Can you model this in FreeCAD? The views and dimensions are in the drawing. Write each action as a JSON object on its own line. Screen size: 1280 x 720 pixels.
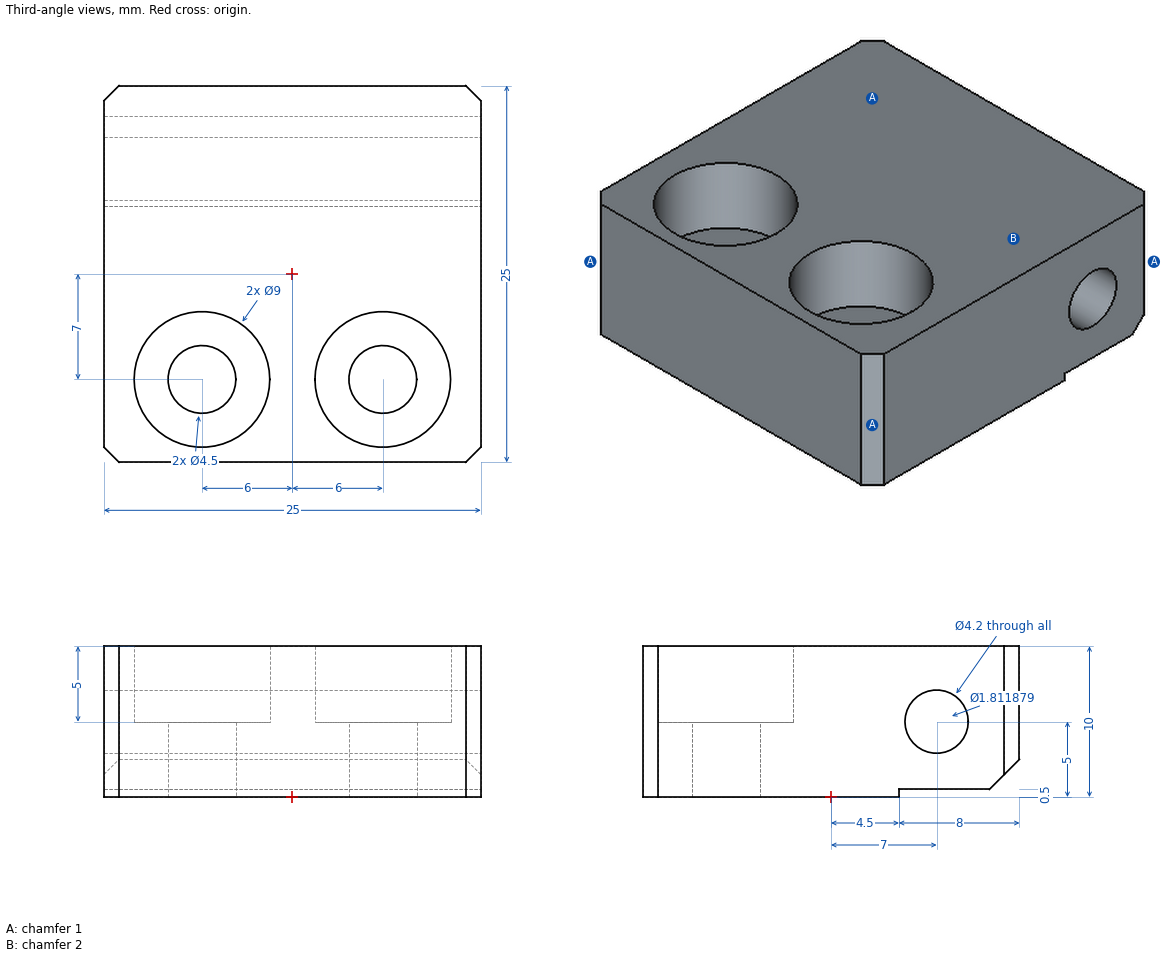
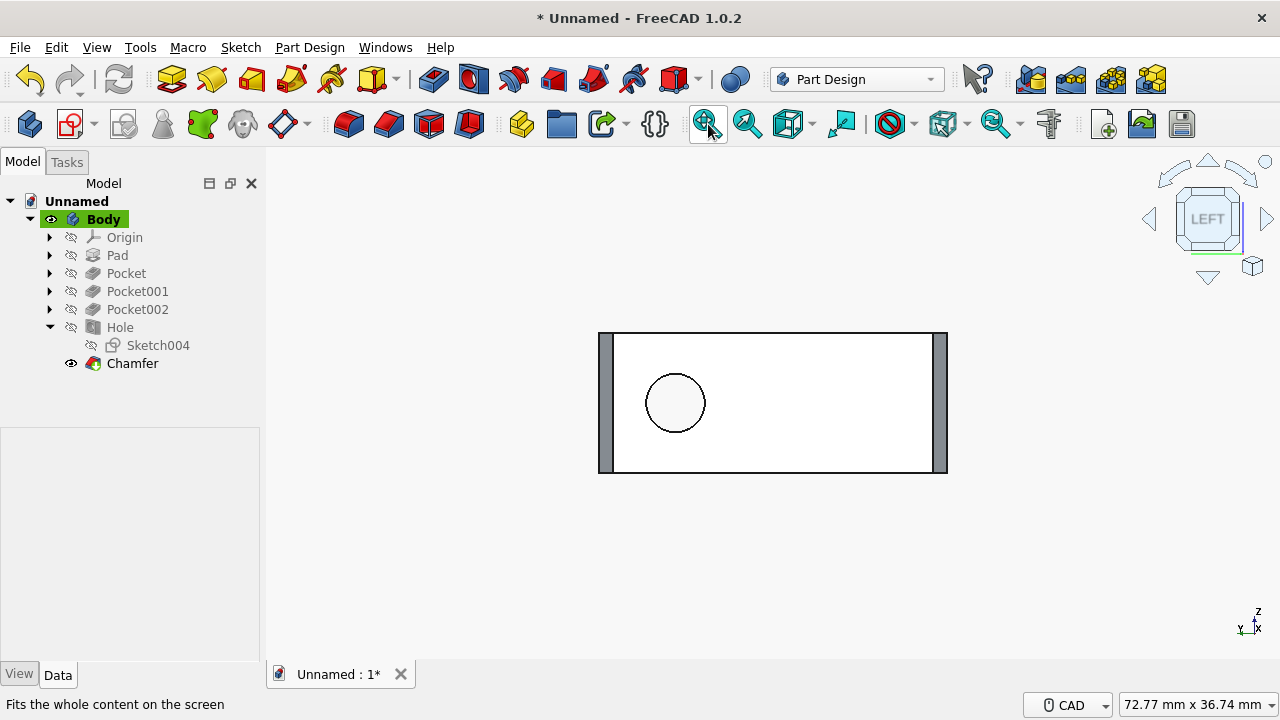
{"action": "left_click", "coordinate": [708, 124]}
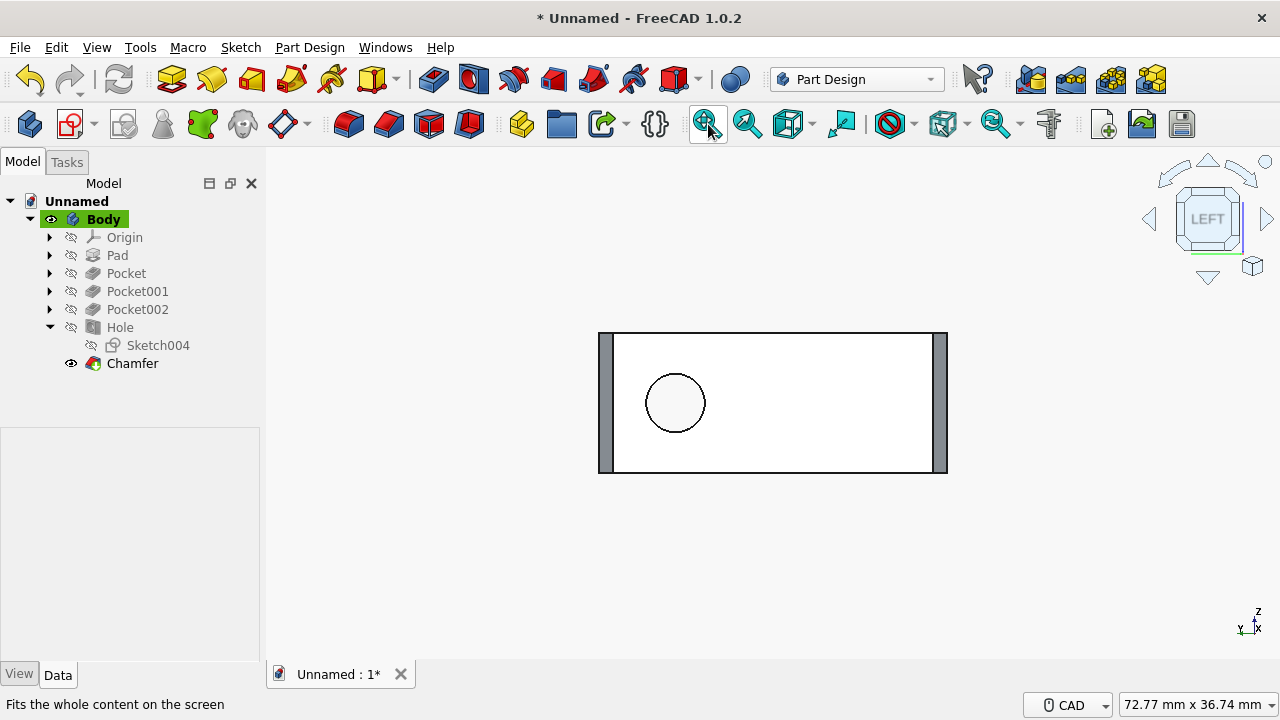
{"action": "left_click", "coordinate": [819, 402]}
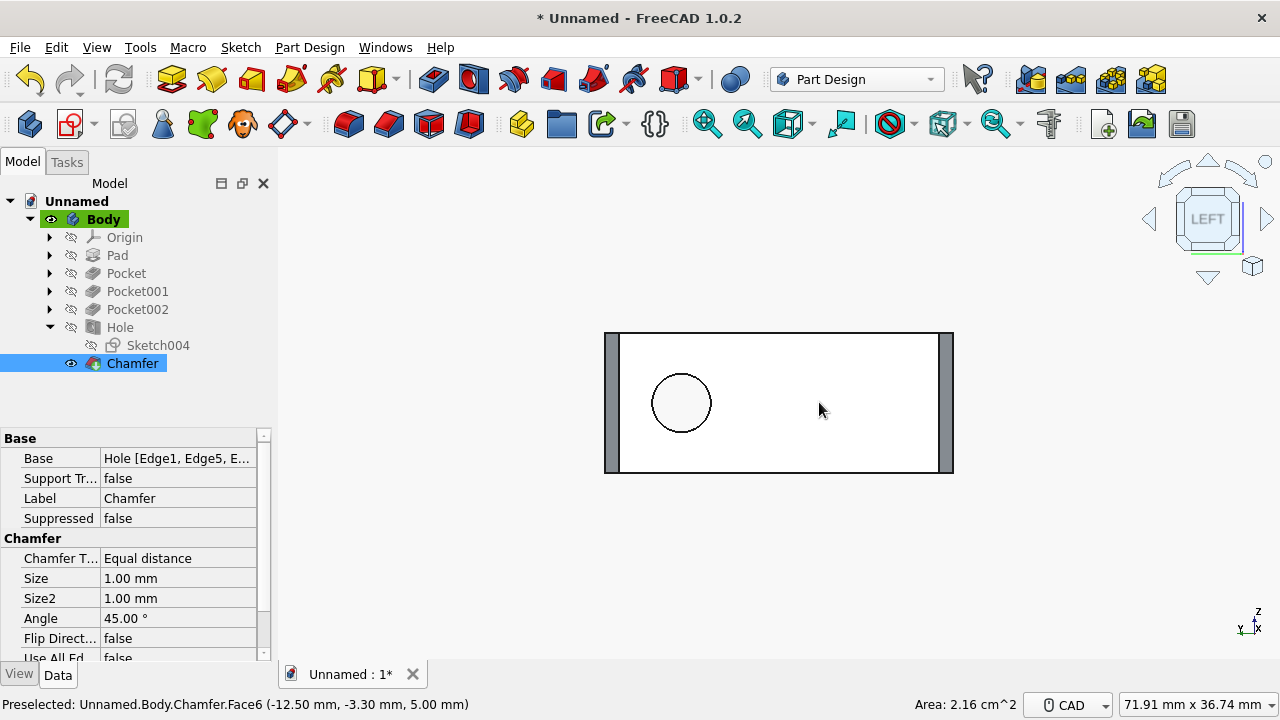
{"action": "left_click", "coordinate": [70, 124]}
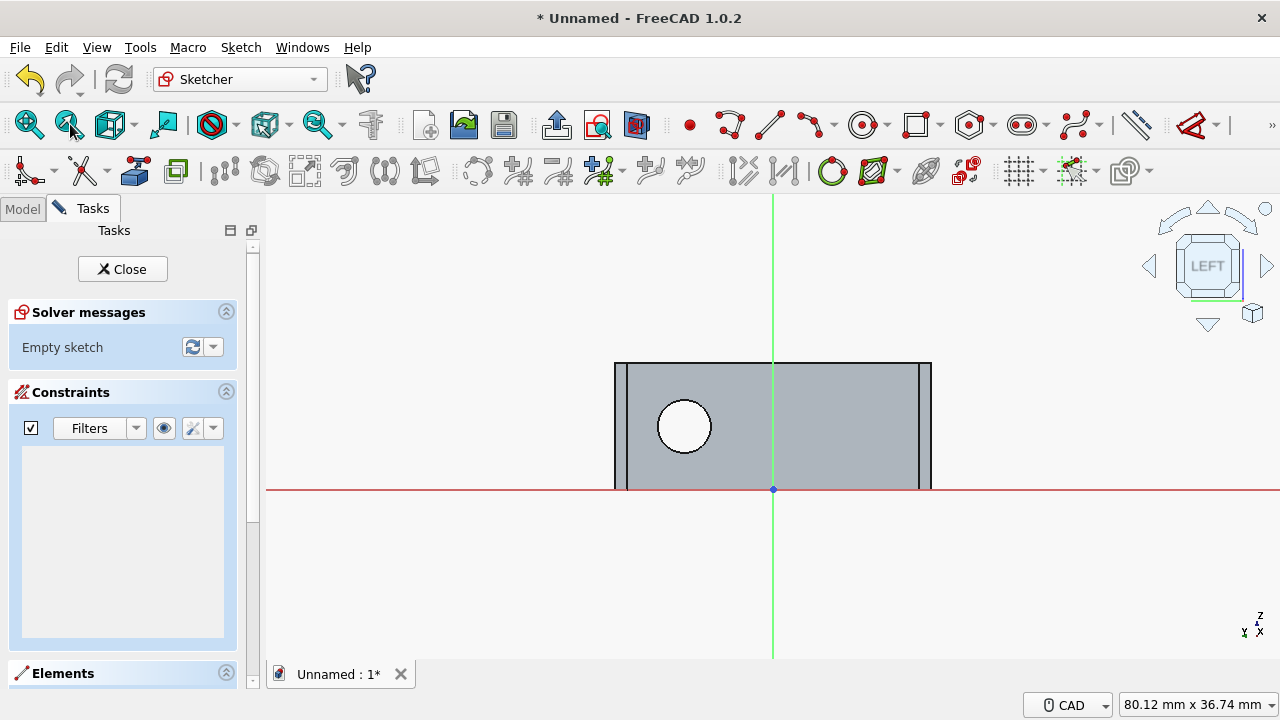
{"action": "scroll", "coordinate": [689, 513], "scroll_direction": "up", "scroll_amount": 6}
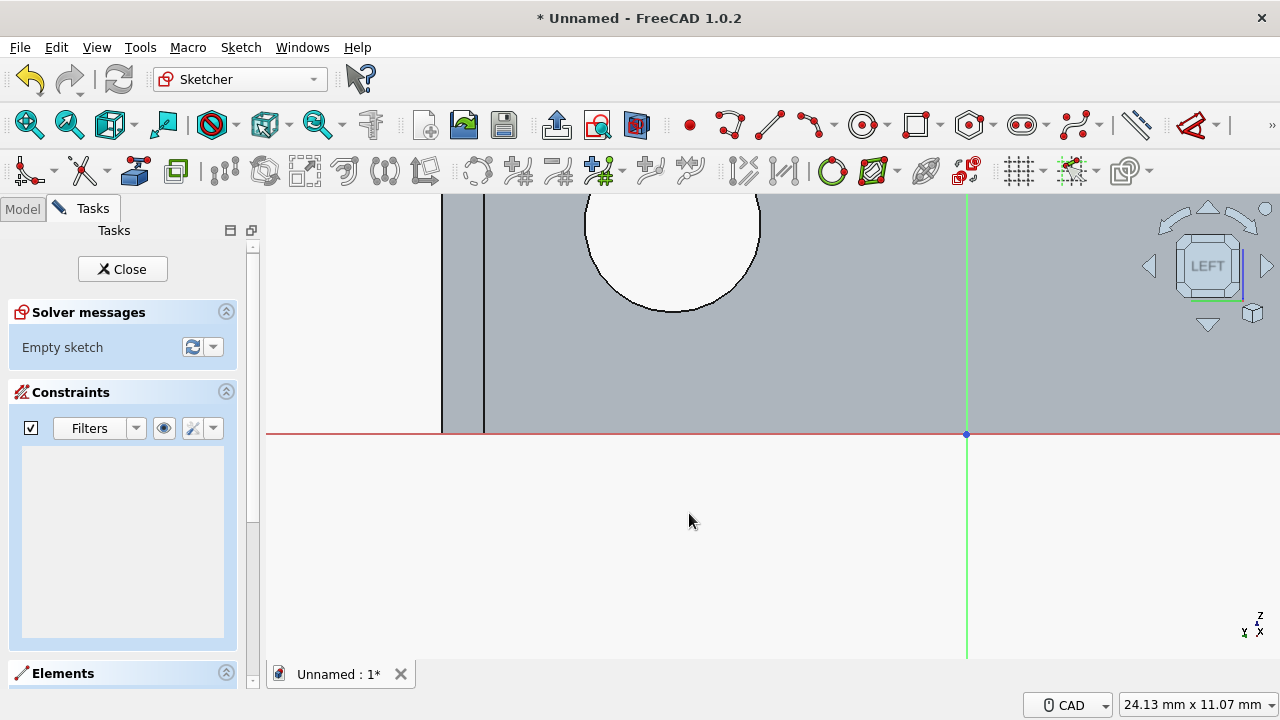
{"action": "left_click", "coordinate": [916, 126]}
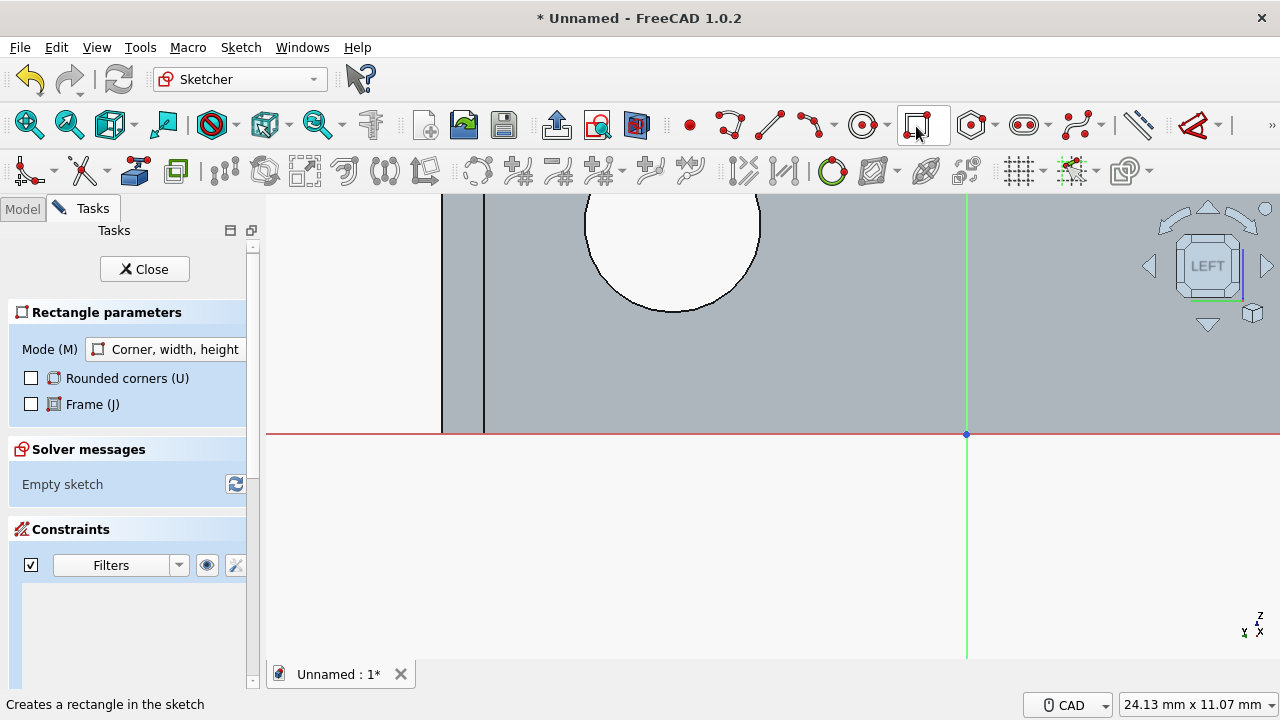
{"action": "left_click", "coordinate": [442, 413]}
{"action": "left_click", "coordinate": [778, 434]}
{"action": "key", "text": "Escape"}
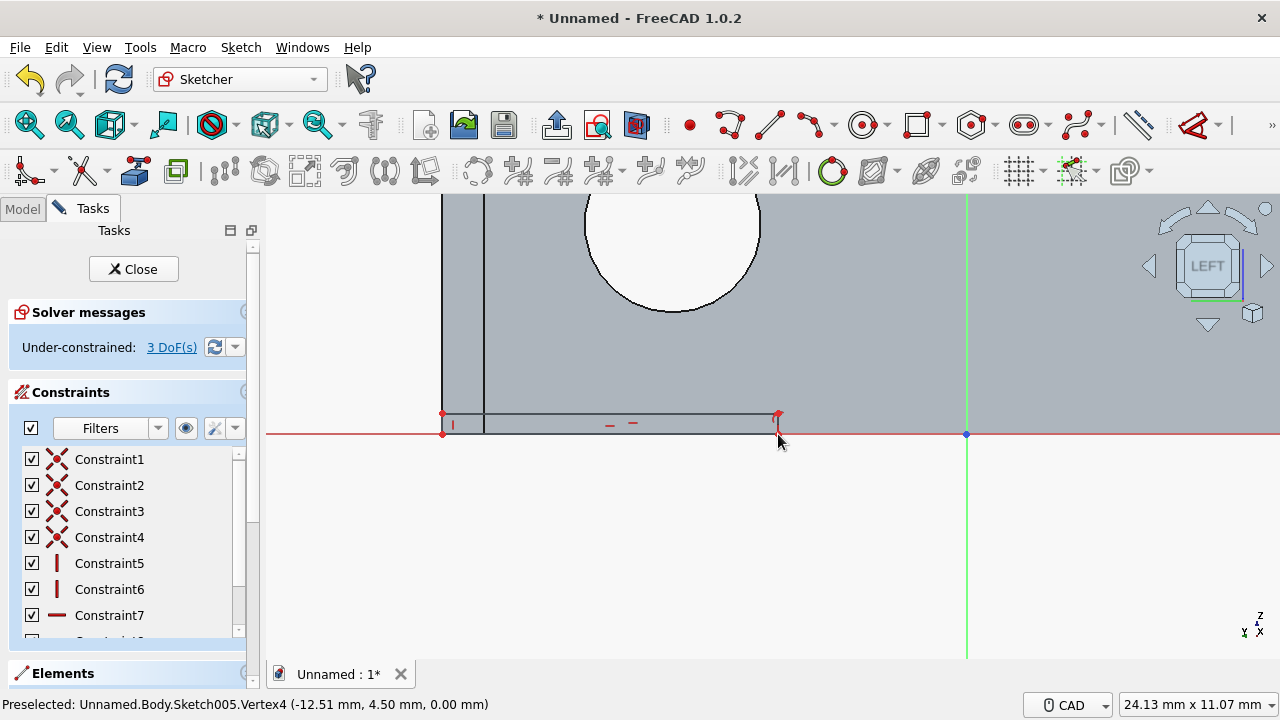
{"action": "key", "text": "d"}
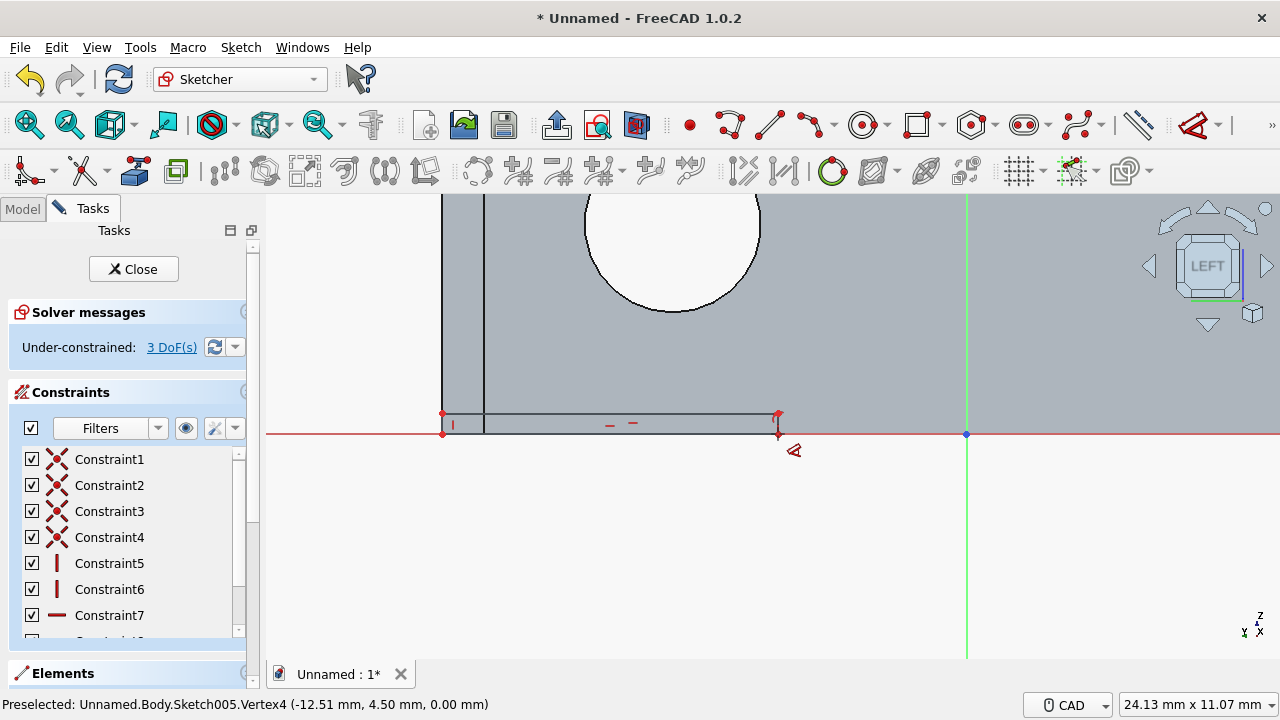
{"action": "left_click", "coordinate": [543, 434]}
{"action": "left_click", "coordinate": [610, 468]}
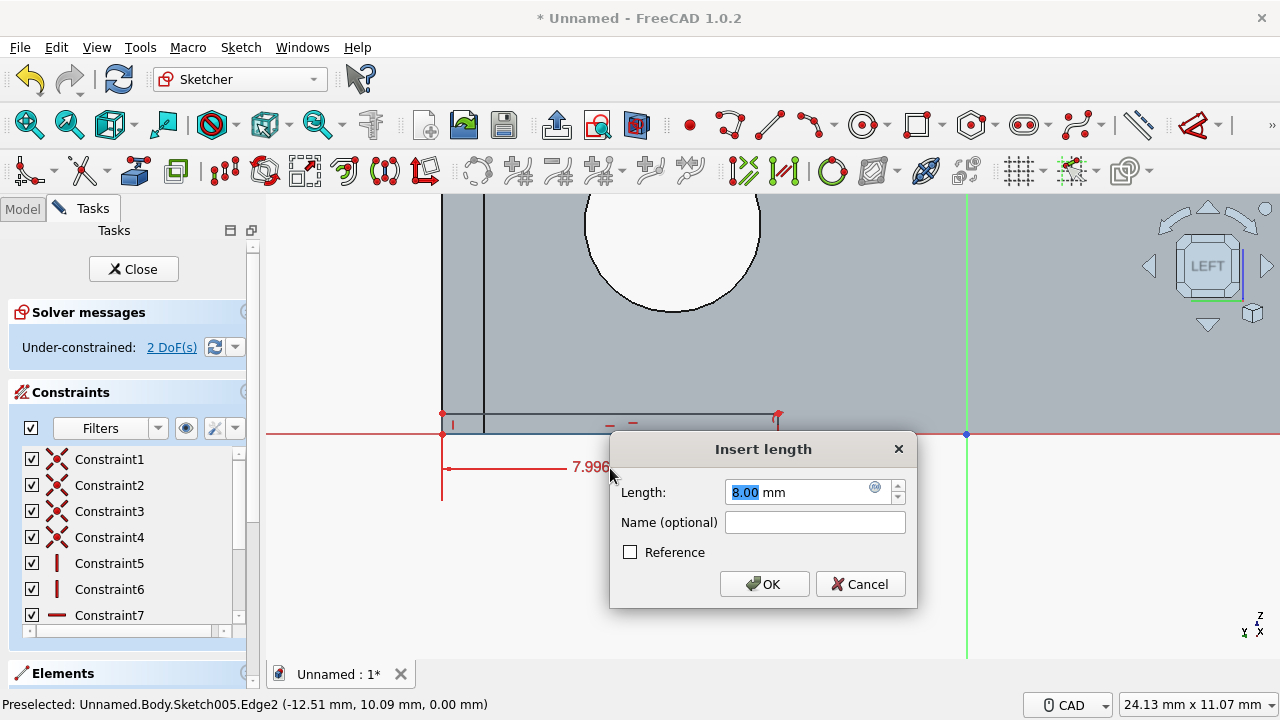
{"action": "type", "text": "8"}
{"action": "key", "text": "Return"}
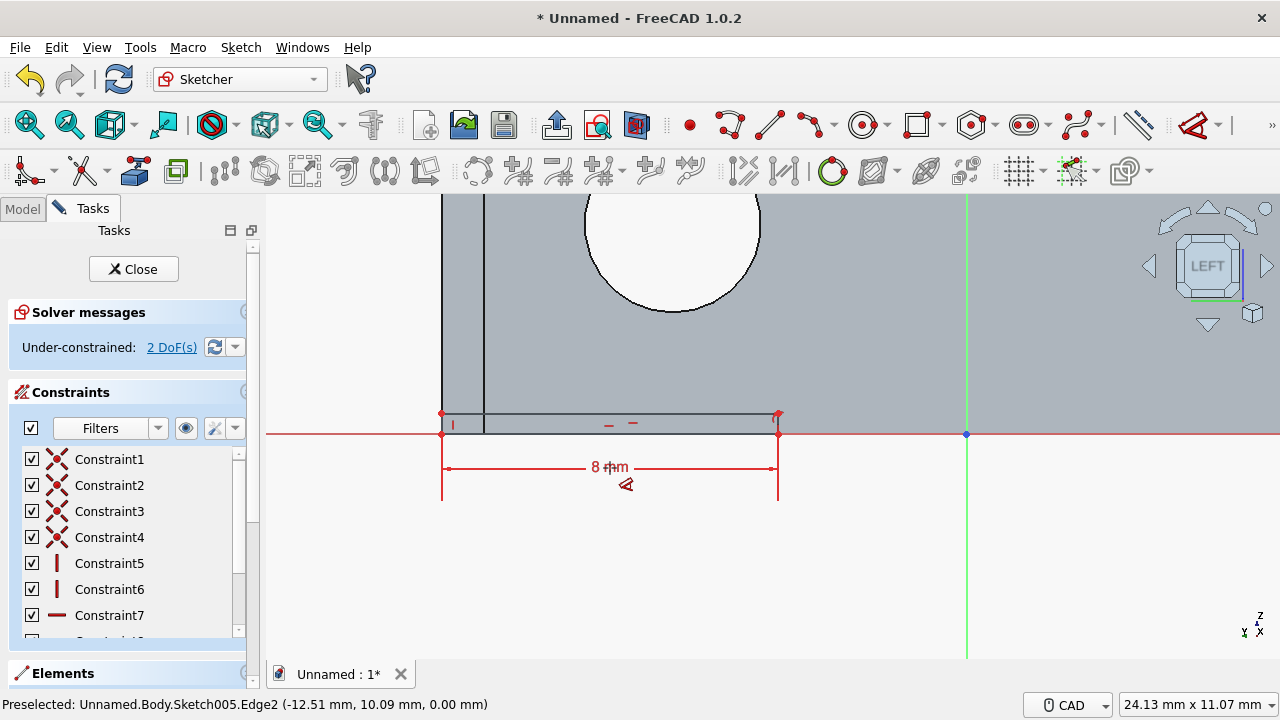
{"action": "scroll", "coordinate": [442, 424], "scroll_direction": "up", "scroll_amount": 4}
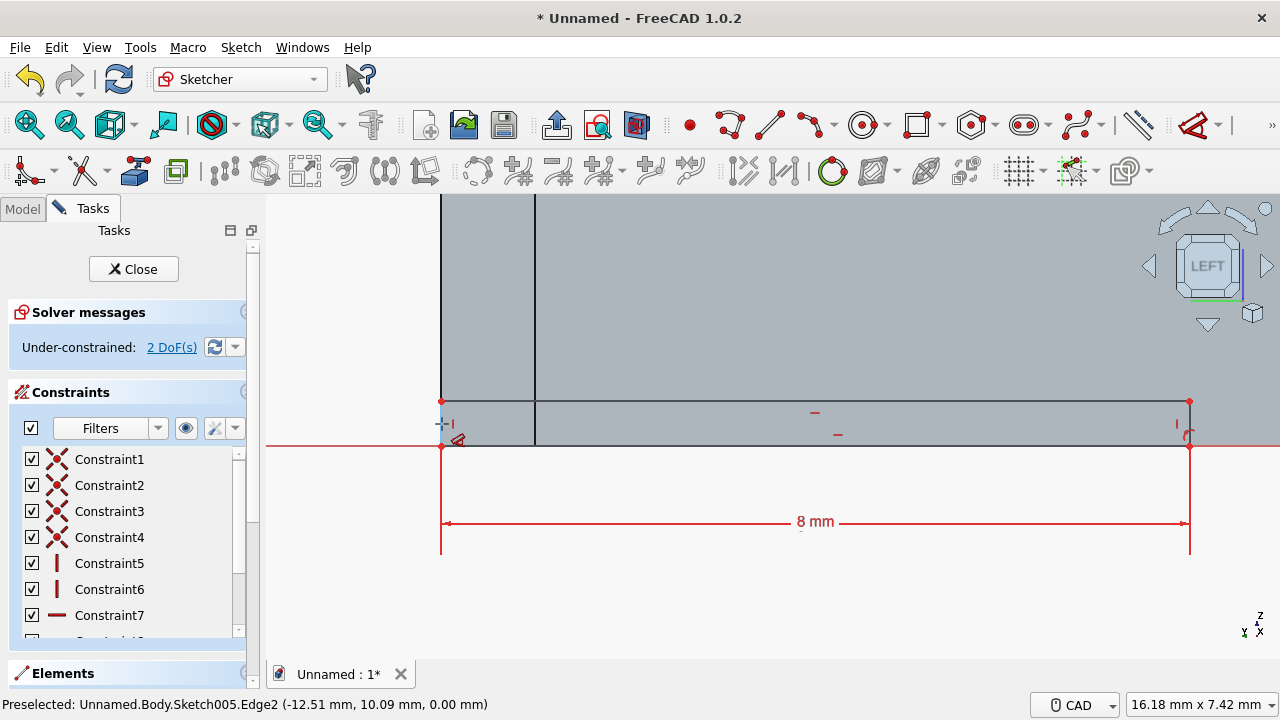
{"action": "left_click", "coordinate": [441, 424]}
{"action": "left_click", "coordinate": [407, 424]}